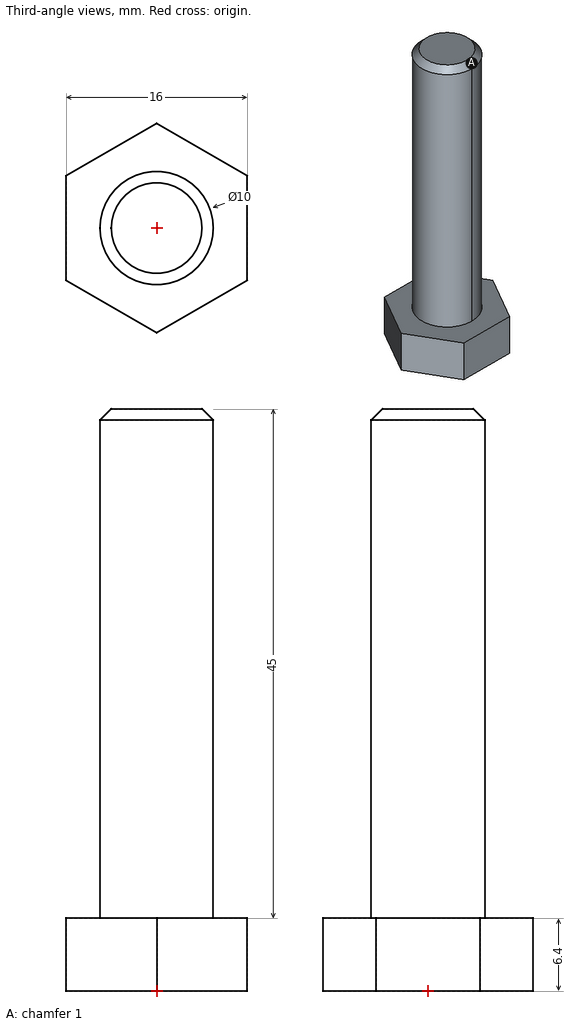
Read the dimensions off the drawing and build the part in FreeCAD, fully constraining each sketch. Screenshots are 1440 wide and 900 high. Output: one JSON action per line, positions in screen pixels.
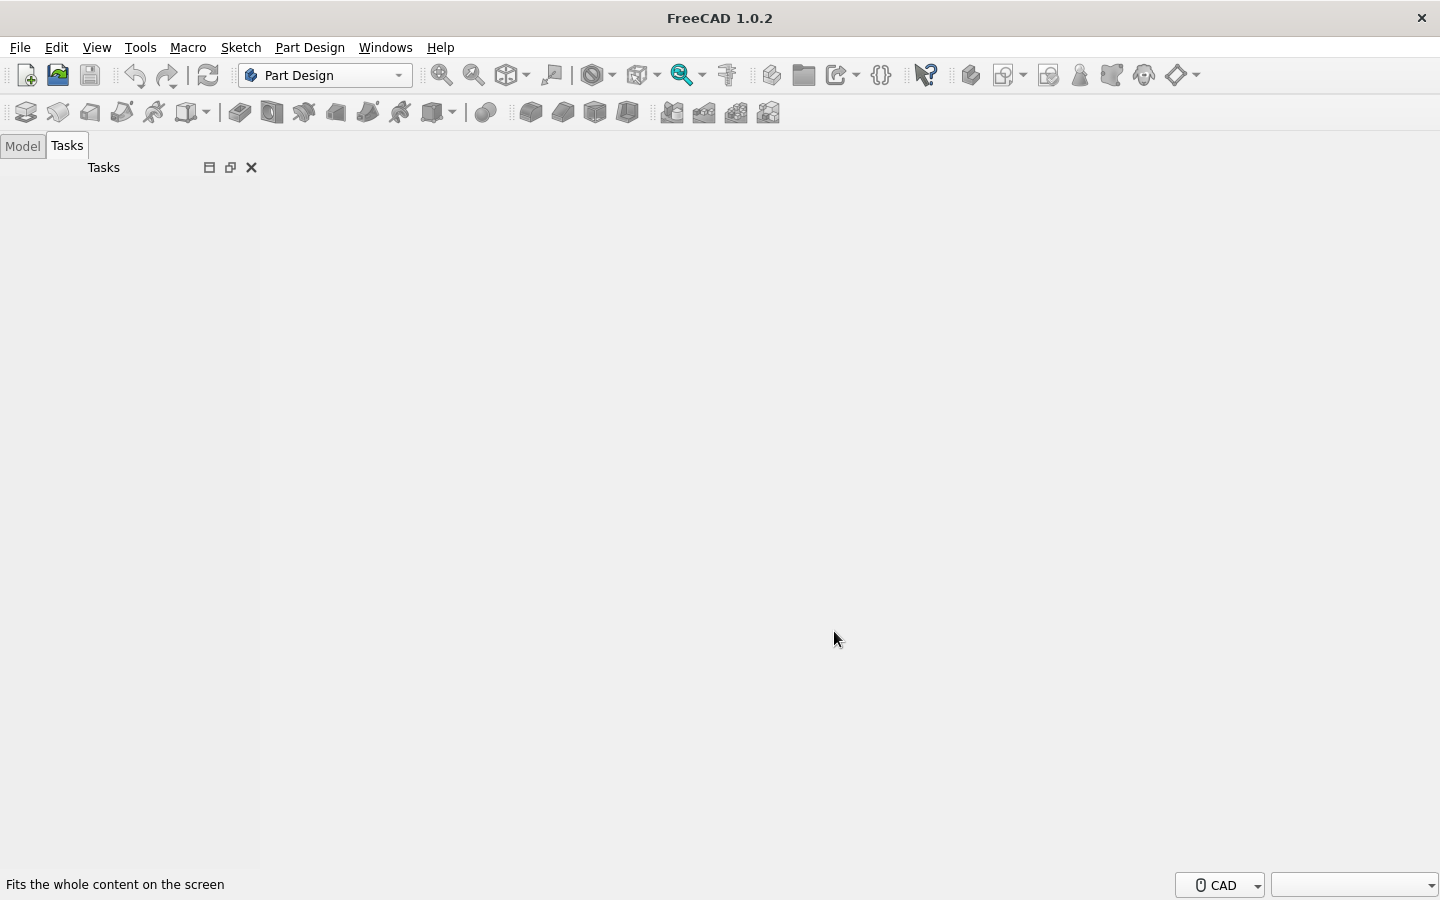
{"action": "left_click", "coordinate": [26, 76]}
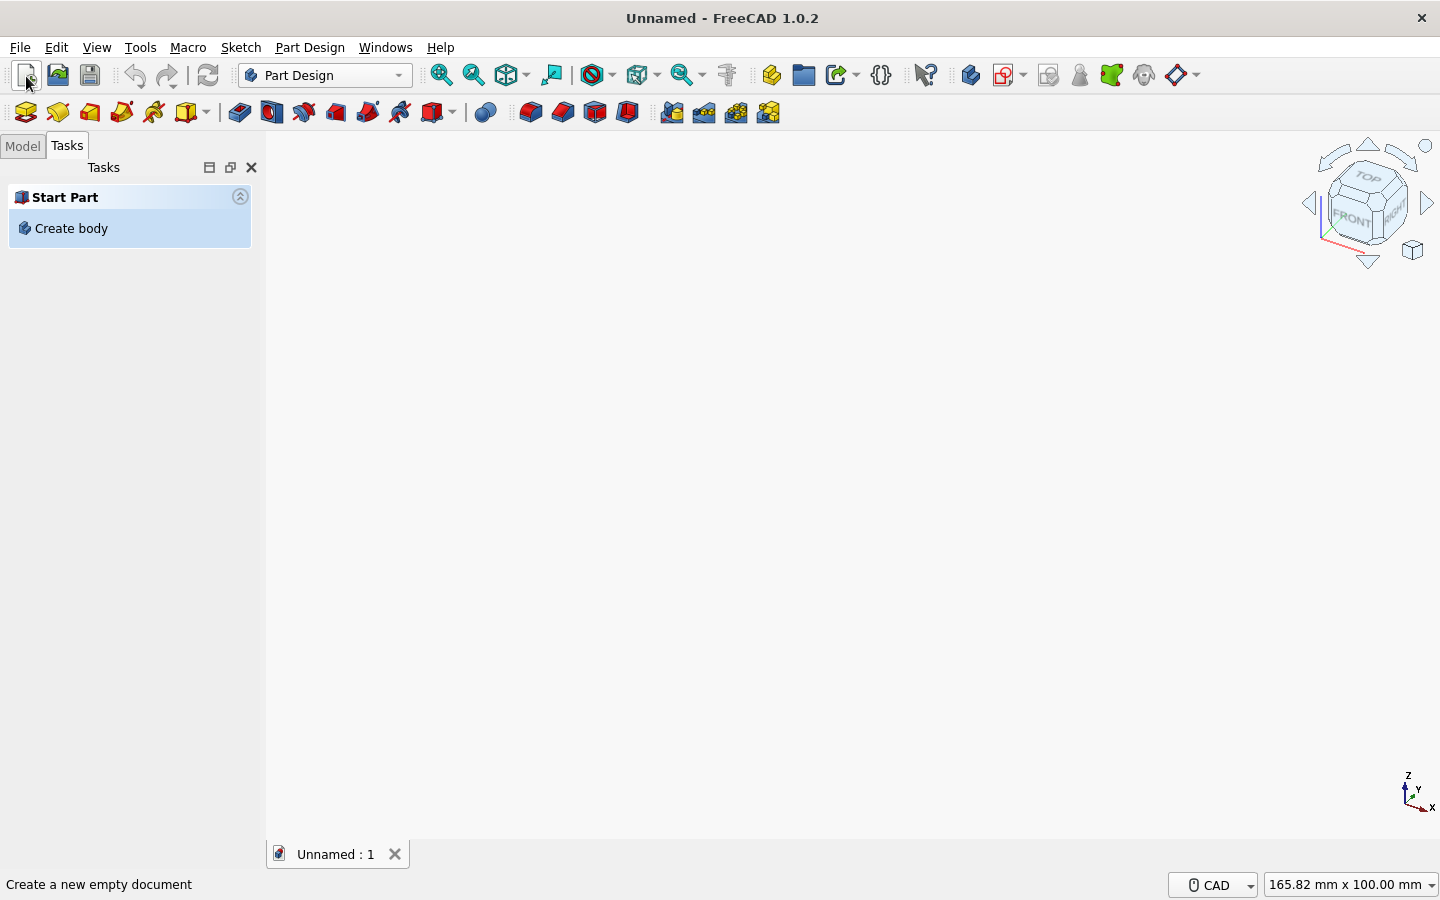
{"action": "left_click", "coordinate": [1004, 76]}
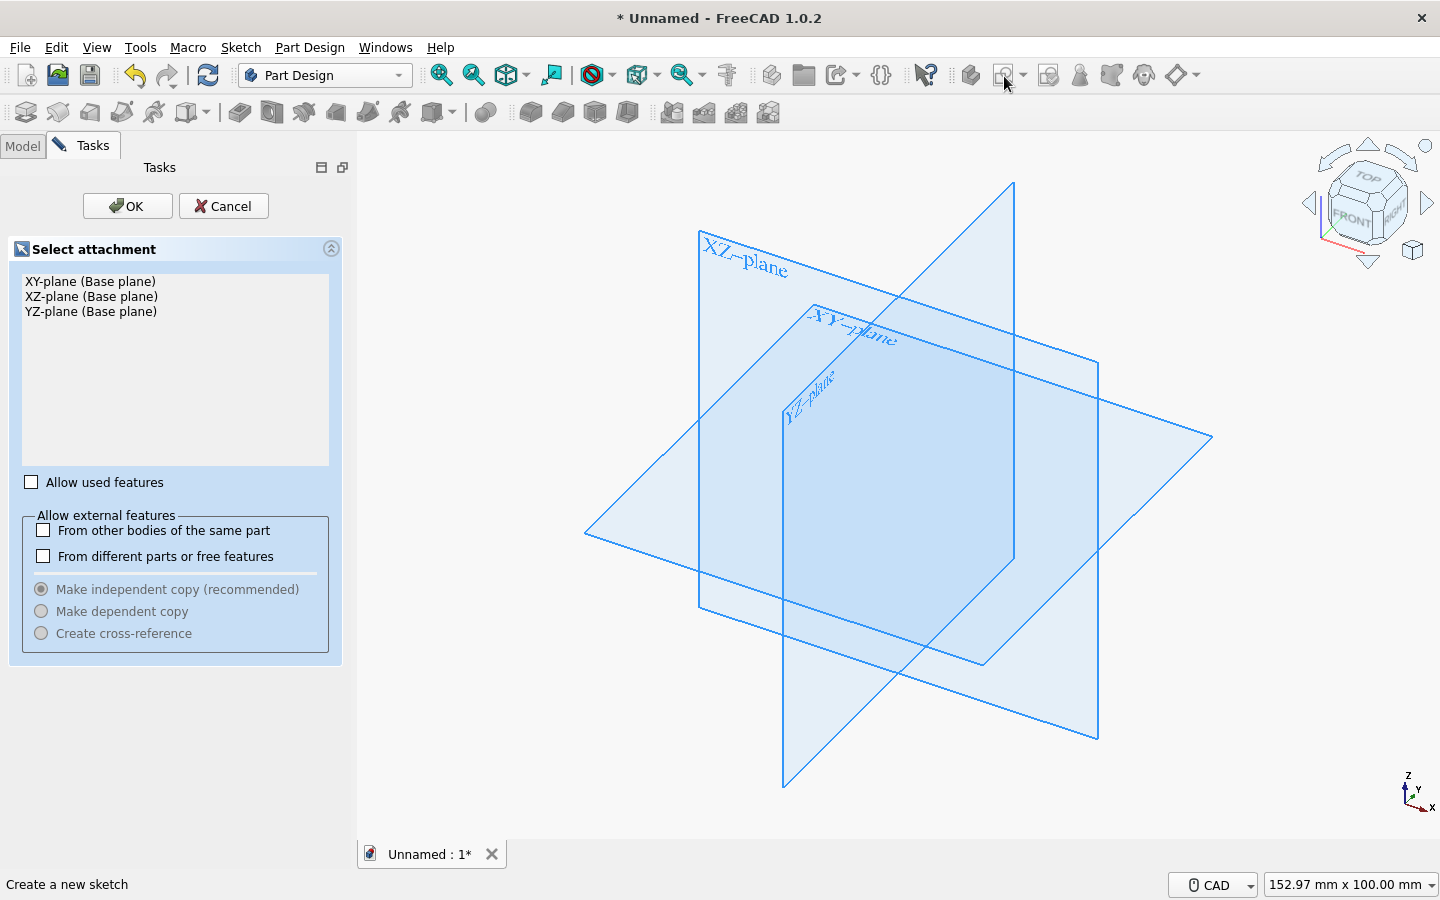
{"action": "left_click", "coordinate": [82, 282]}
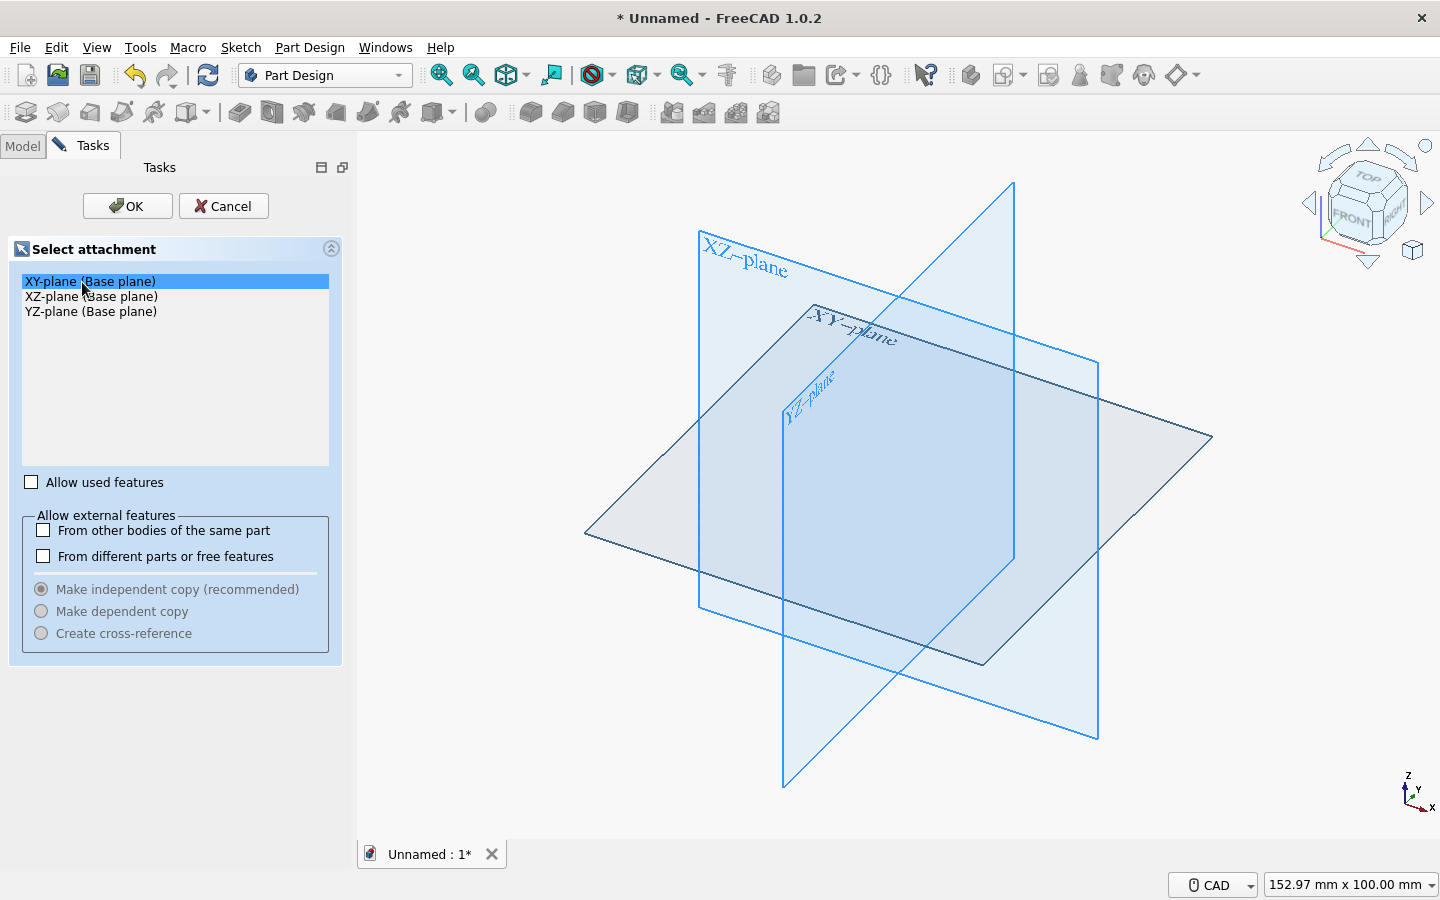
{"action": "left_click", "coordinate": [128, 206]}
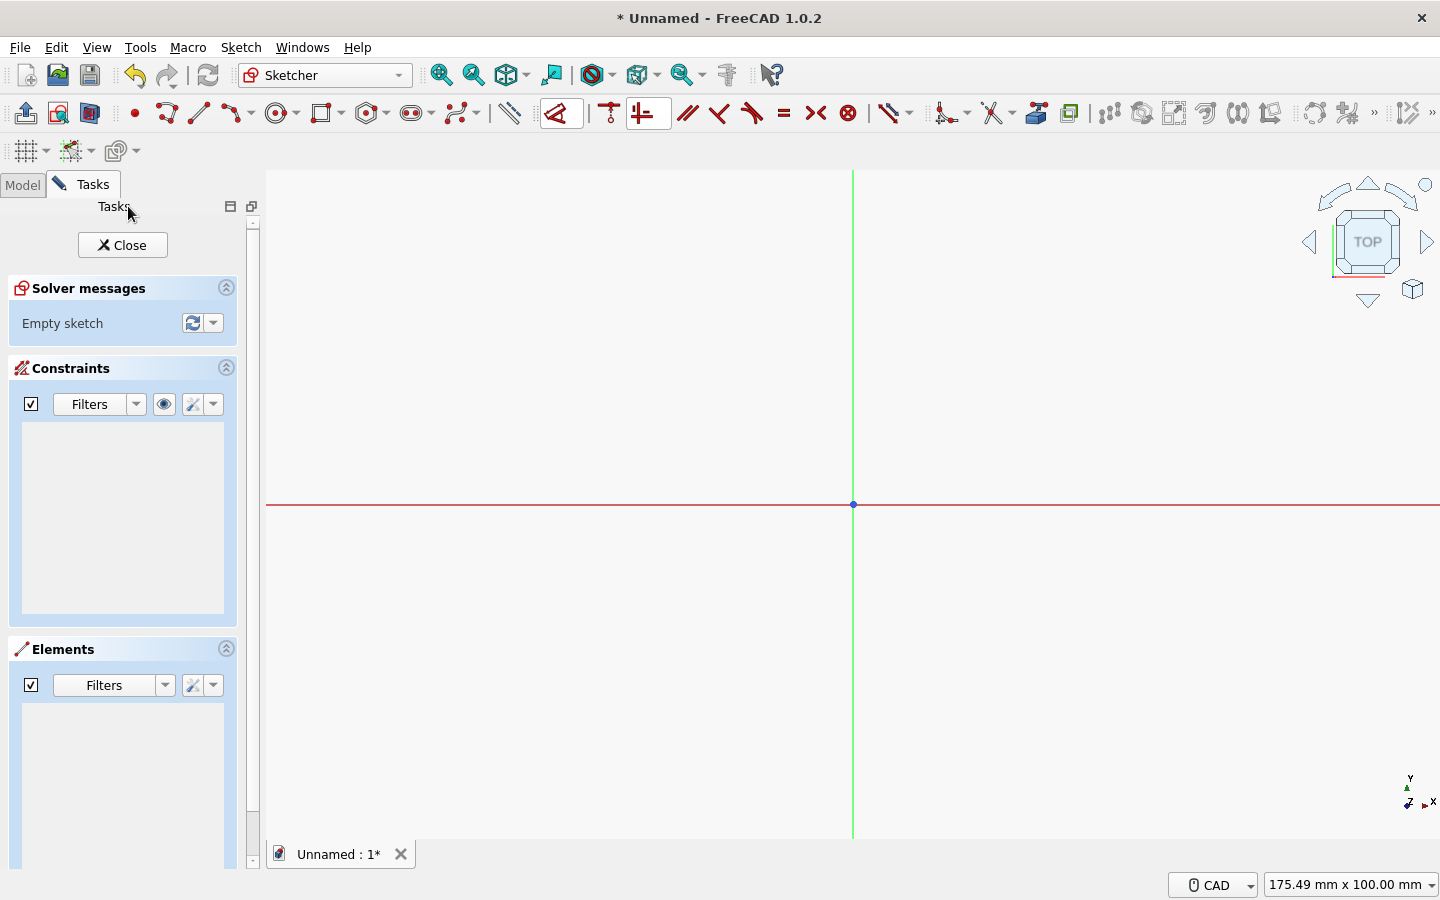
{"action": "scroll", "coordinate": [883, 504], "scroll_direction": "up", "scroll_amount": 6}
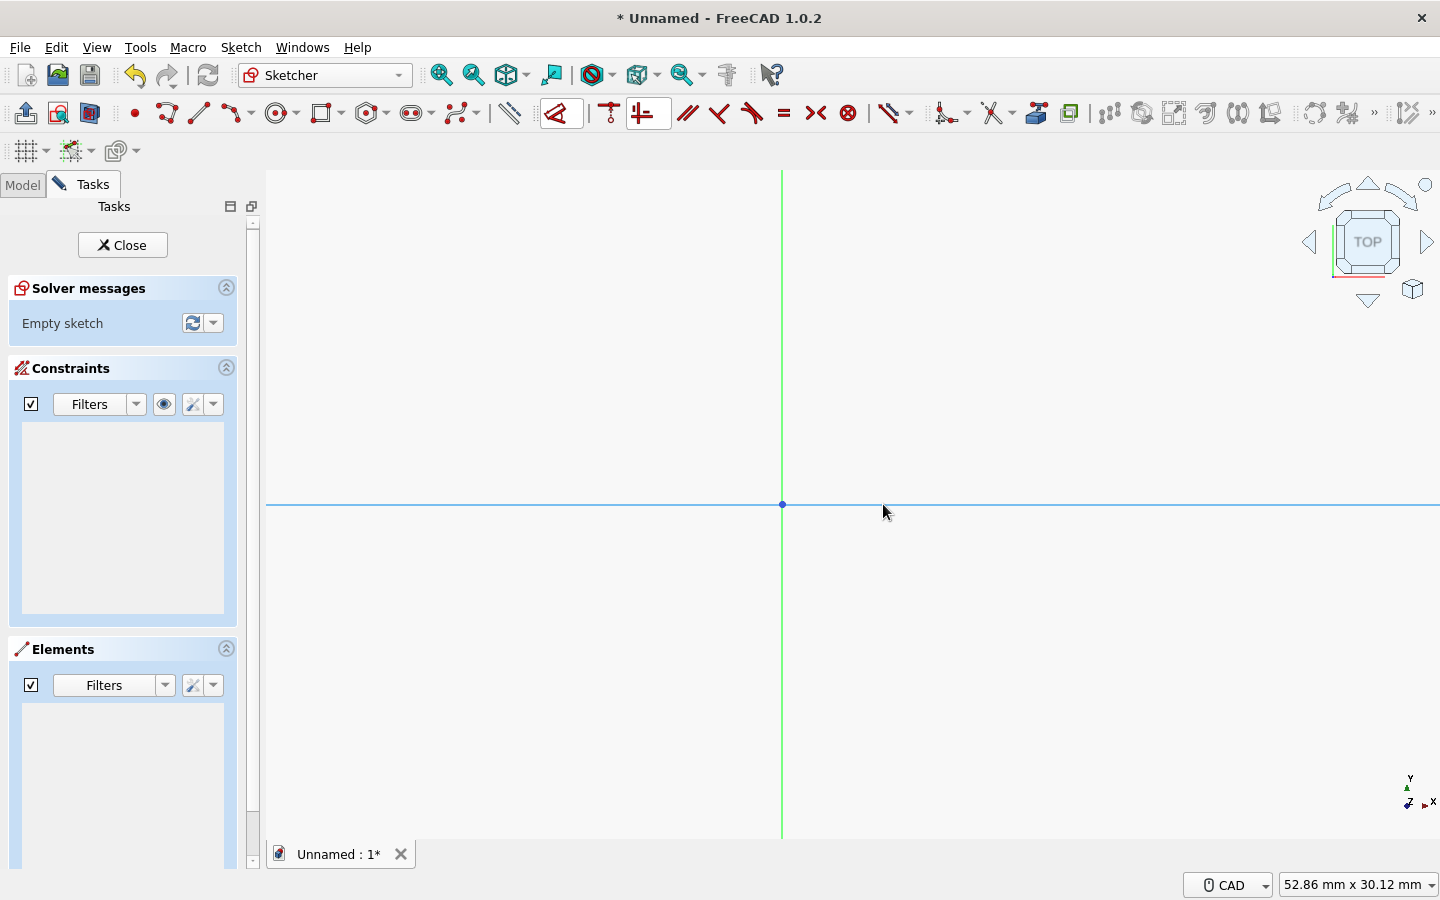
{"action": "left_click", "coordinate": [366, 114]}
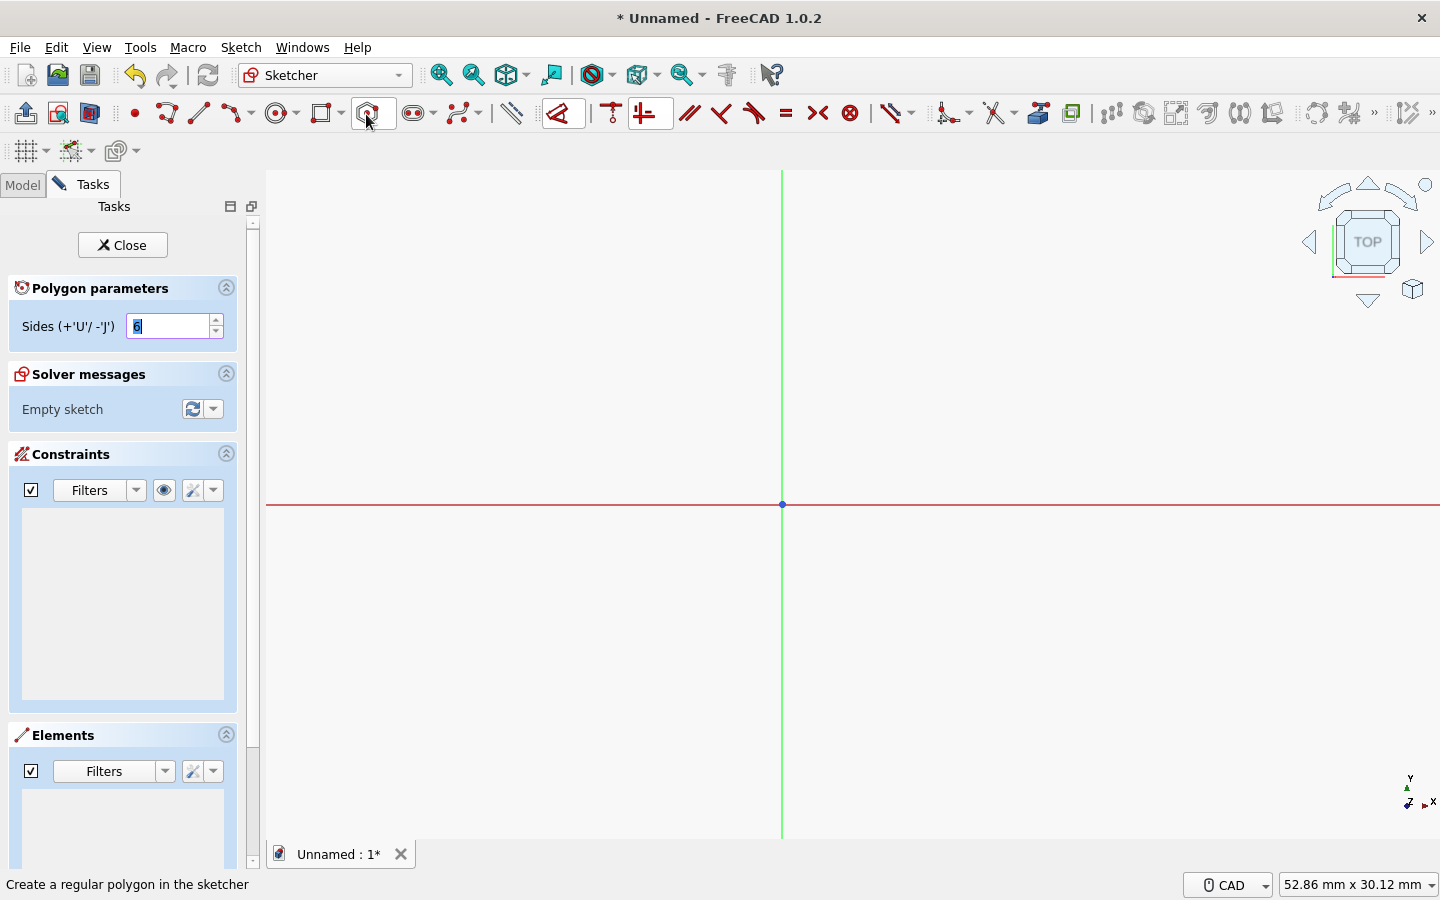
{"action": "left_click", "coordinate": [782, 504]}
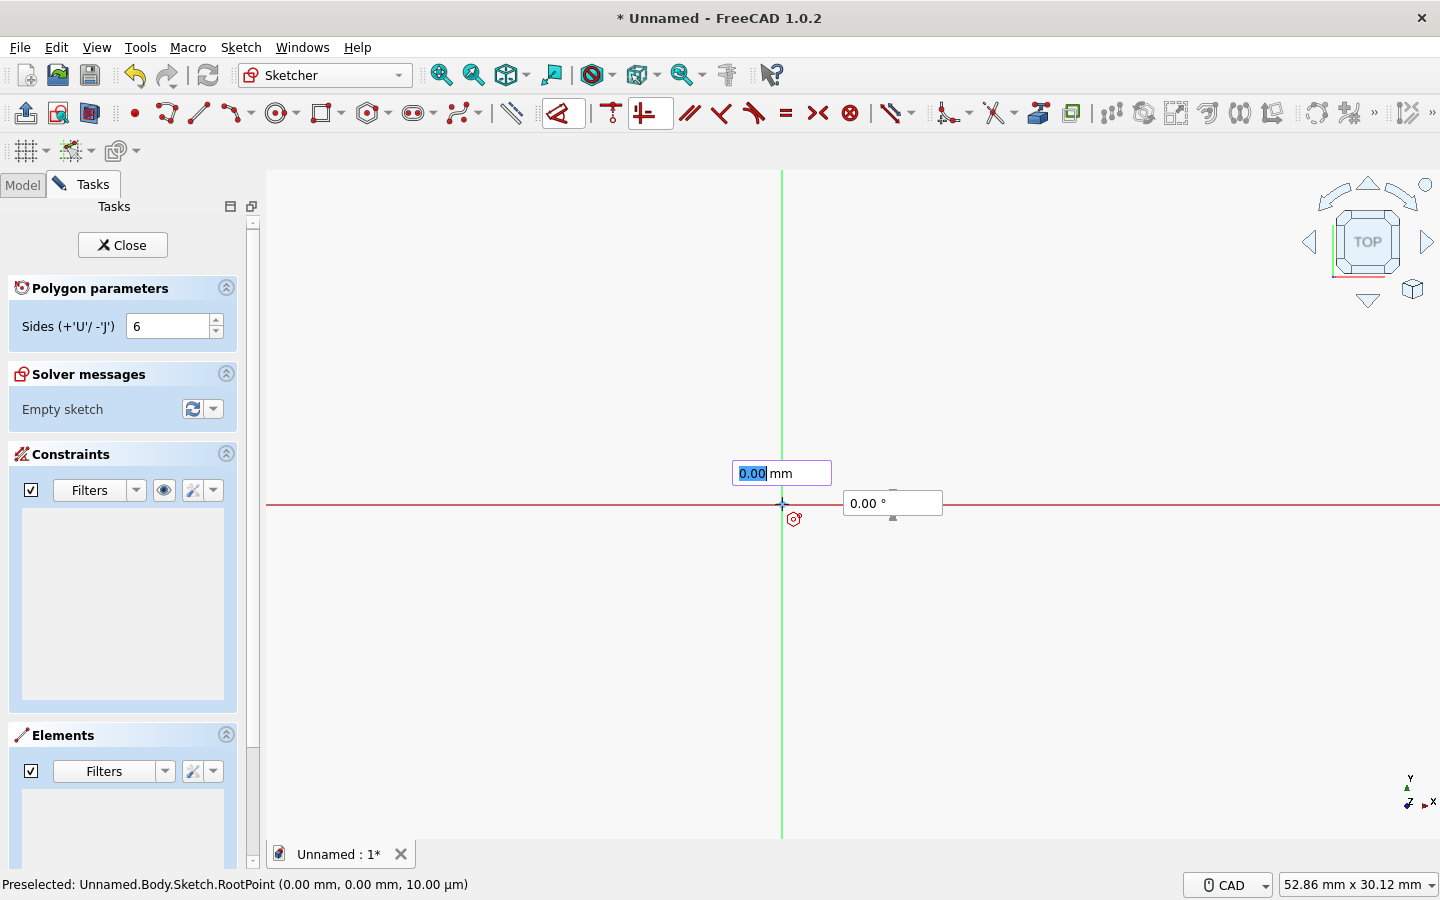
{"action": "left_click", "coordinate": [782, 299]}
{"action": "right_click", "coordinate": [782, 299]}